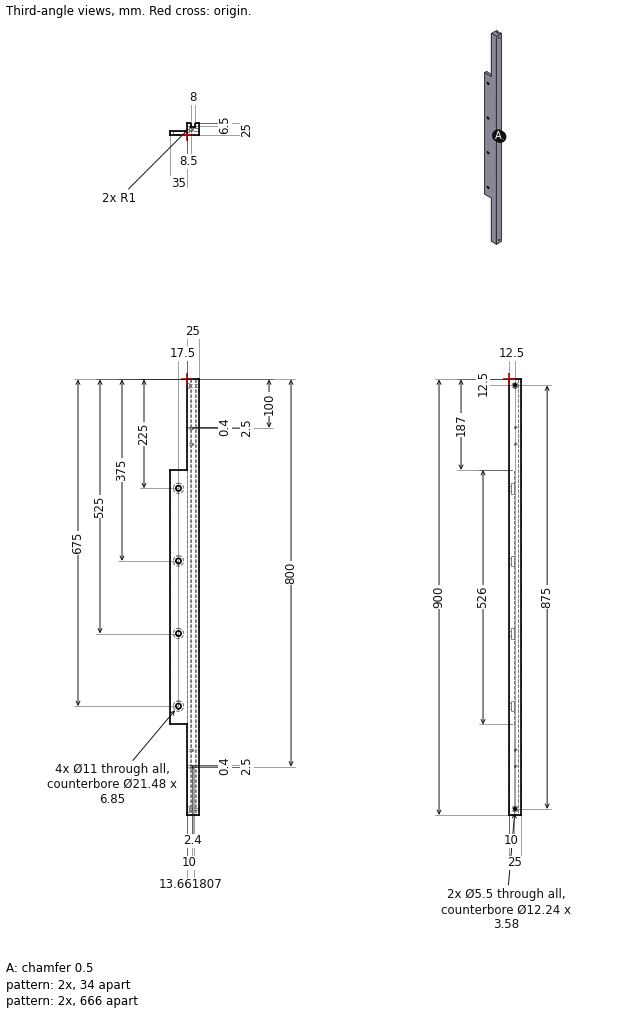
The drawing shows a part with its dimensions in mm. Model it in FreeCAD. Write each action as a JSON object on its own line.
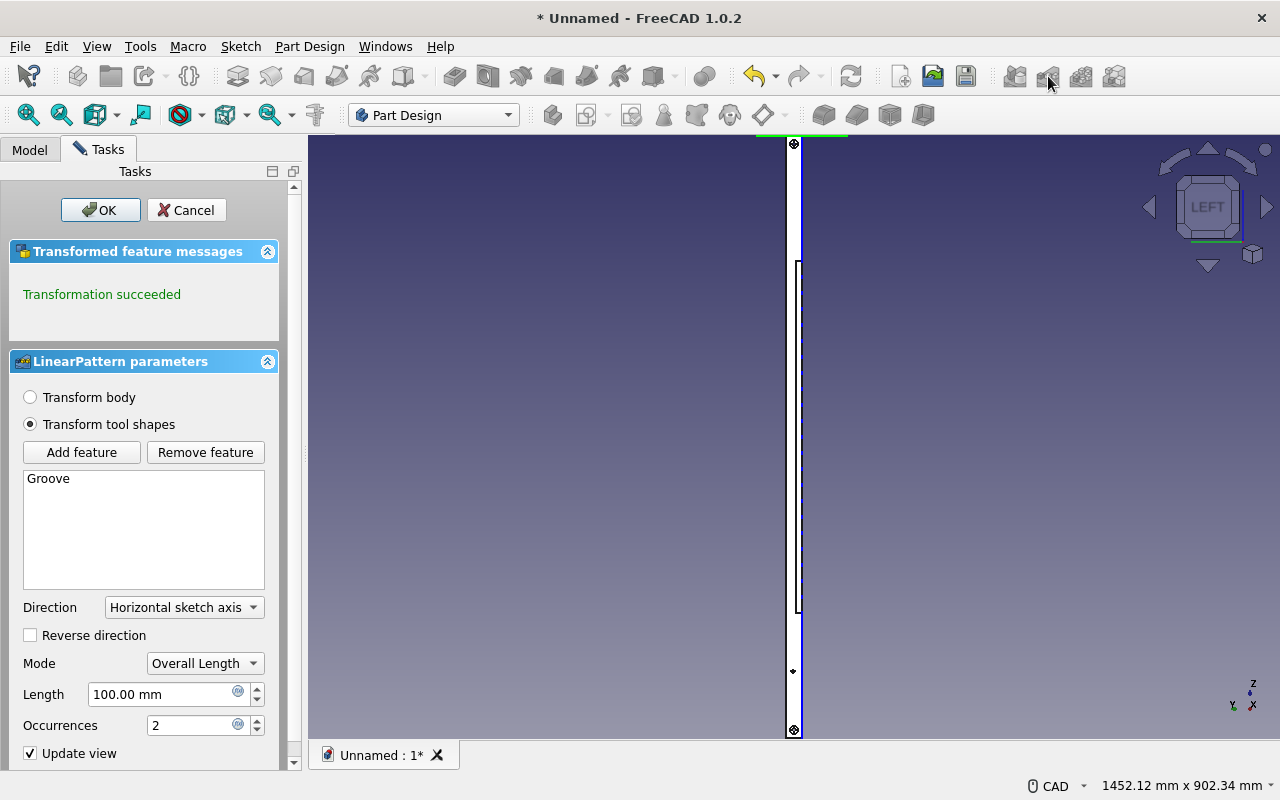
{"action": "left_click", "coordinate": [185, 608]}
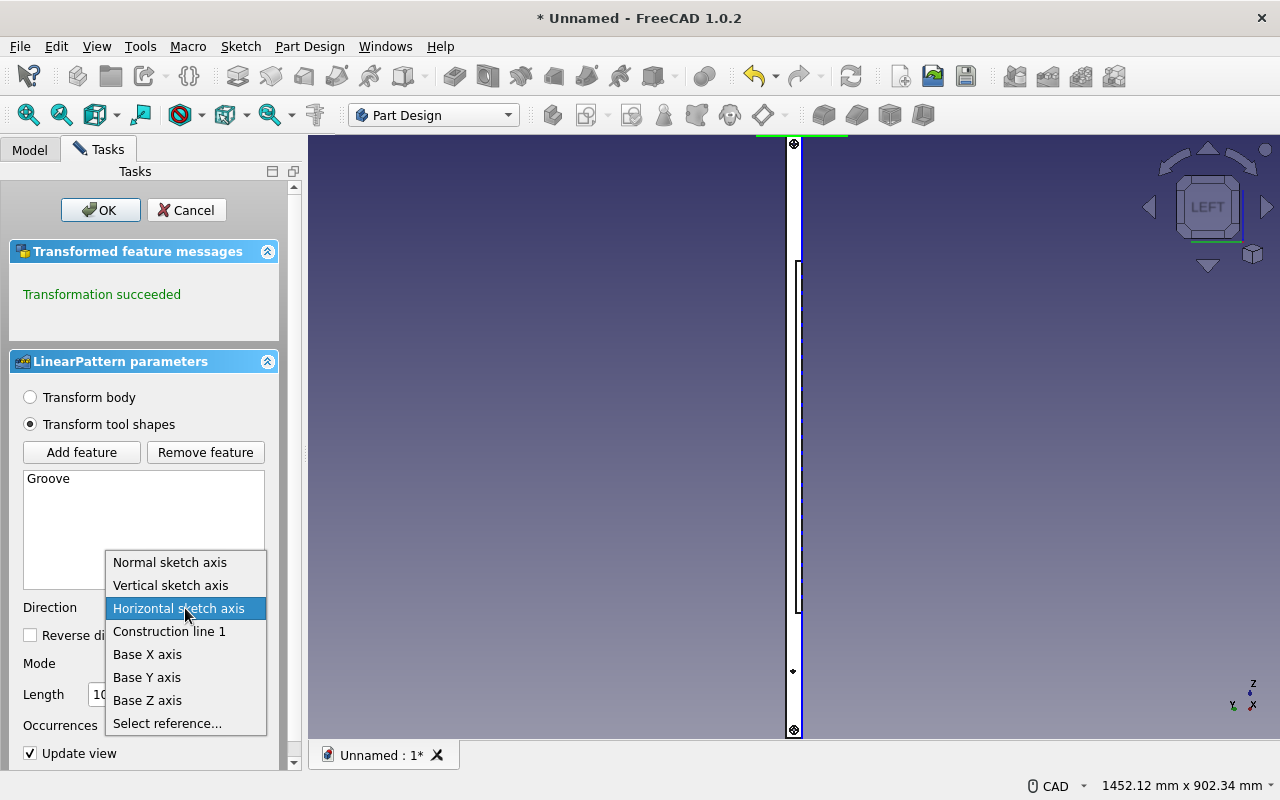
{"action": "left_click", "coordinate": [184, 700]}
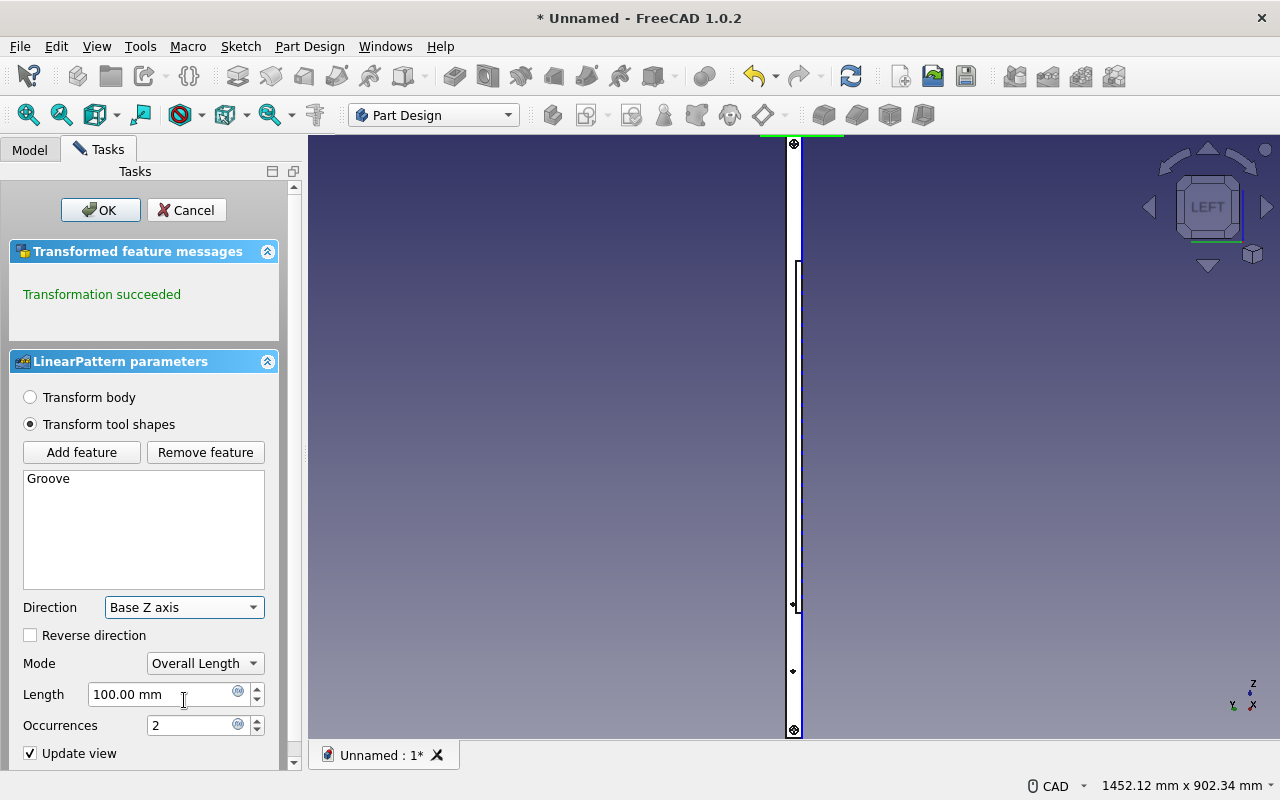
{"action": "left_click", "coordinate": [206, 664]}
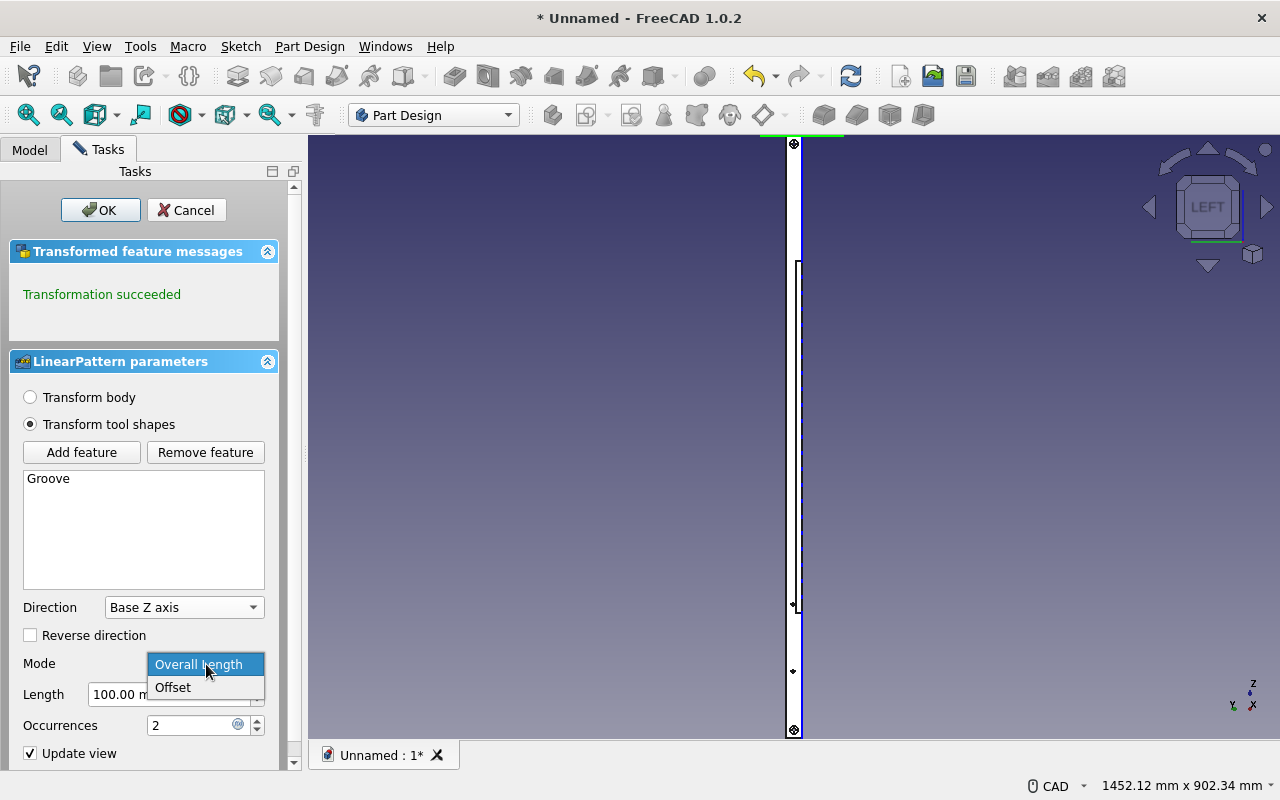
{"action": "left_click", "coordinate": [204, 688]}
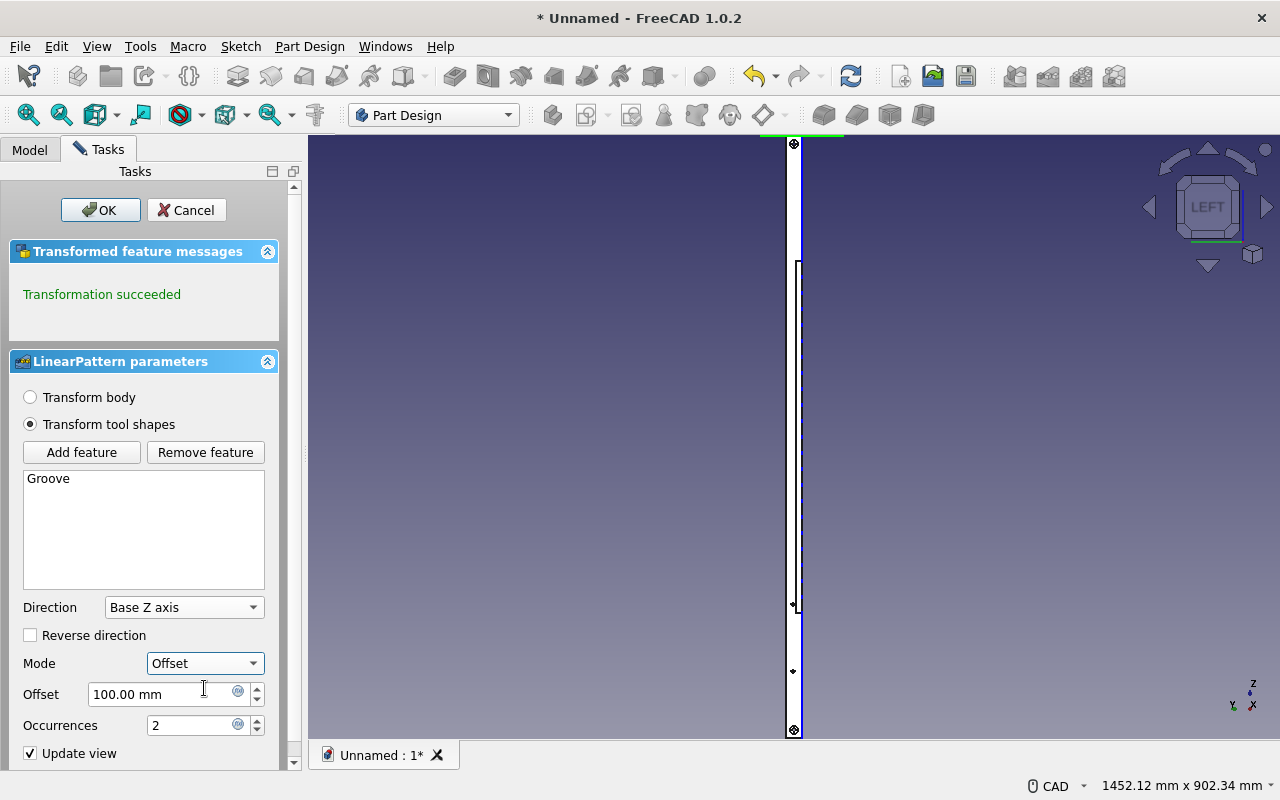
{"action": "triple_click", "coordinate": [170, 694]}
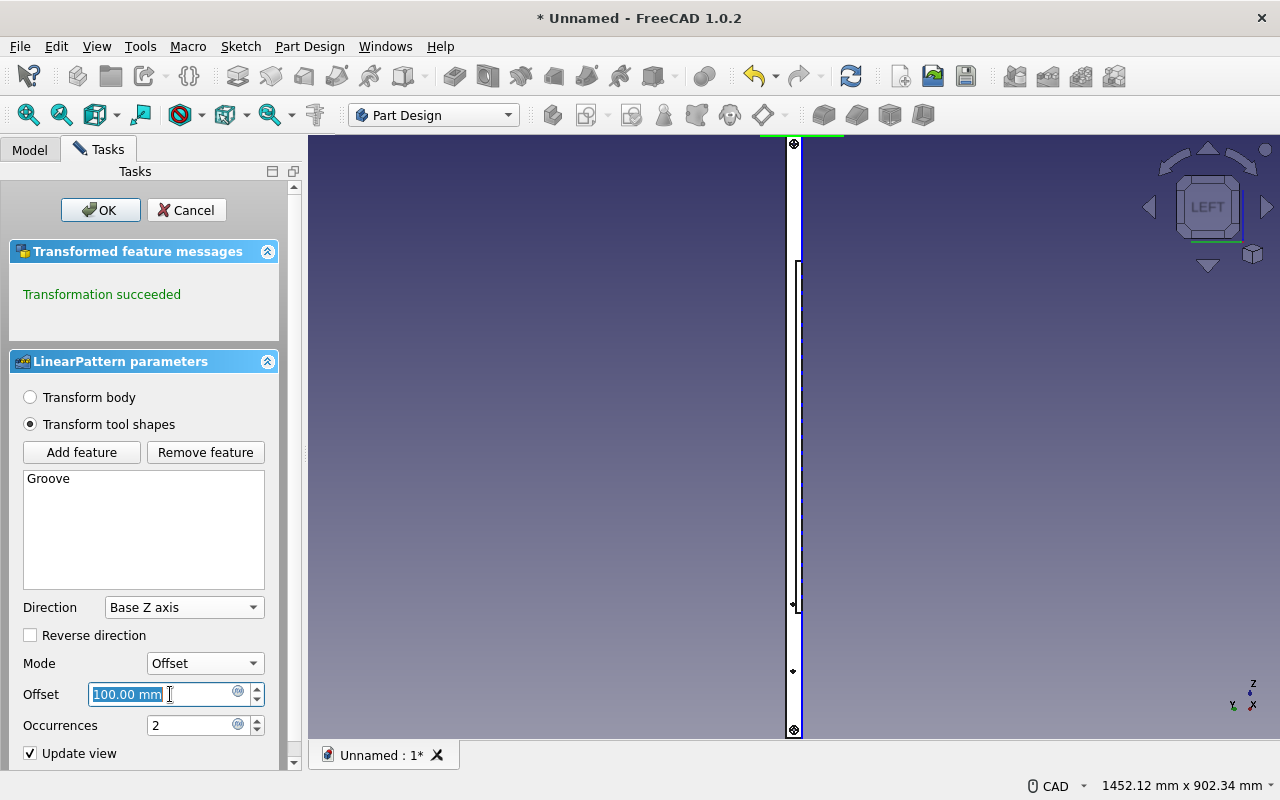
{"action": "type", "text": "34"}
{"action": "key", "text": "Tab"}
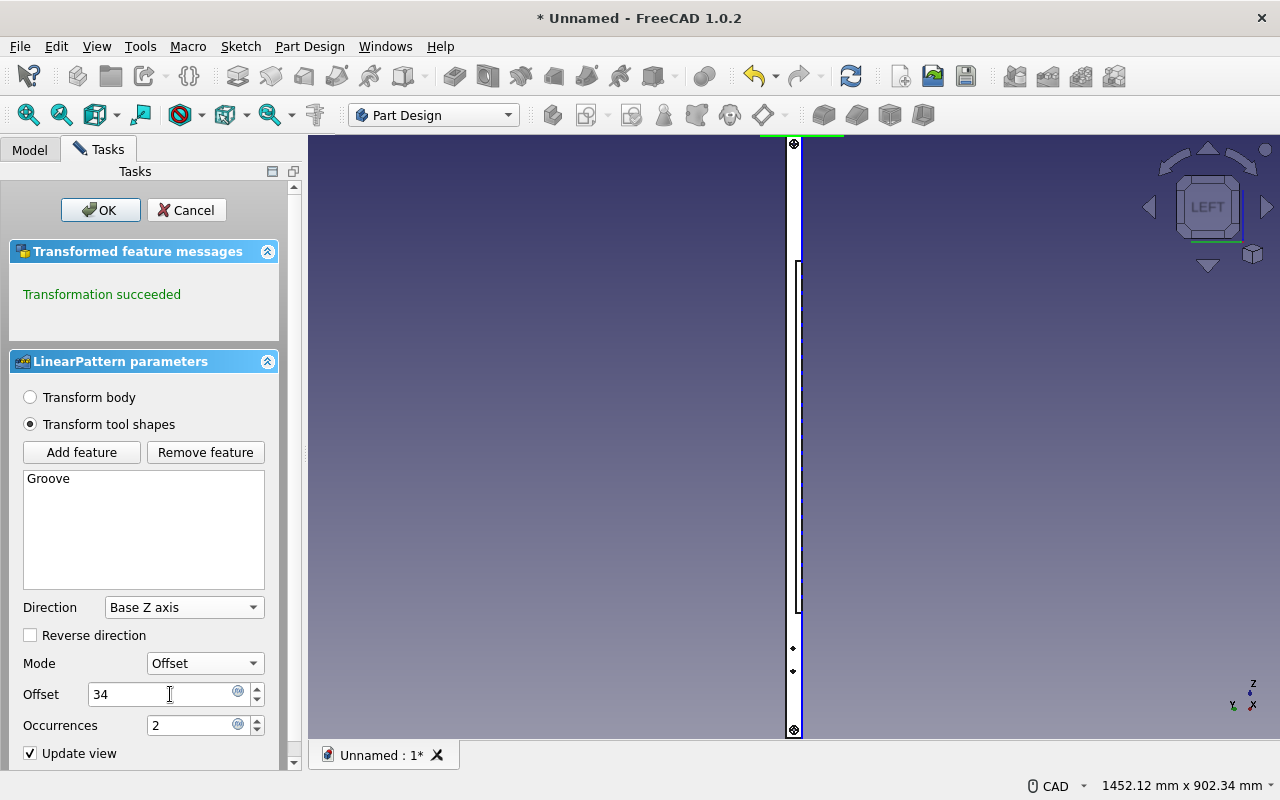
{"action": "triple_click", "coordinate": [199, 726]}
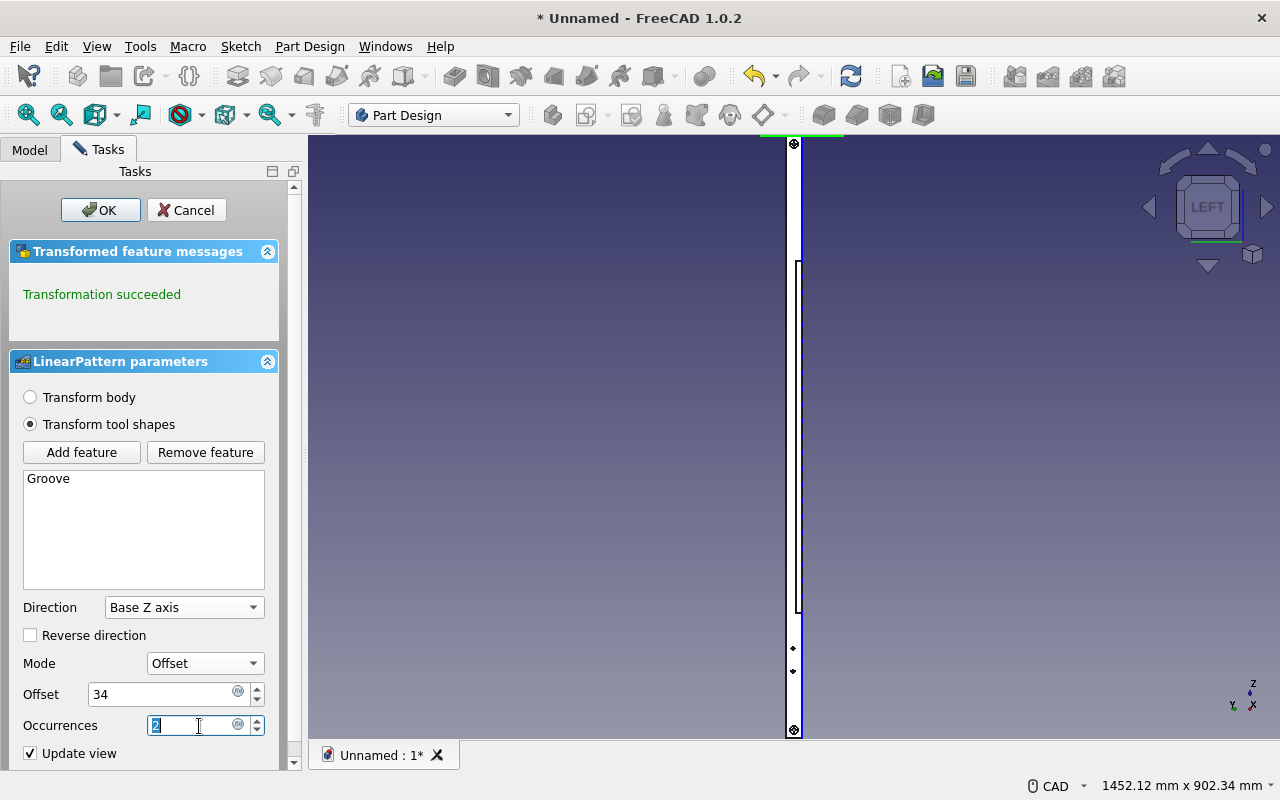
{"action": "type", "text": "2"}
{"action": "key", "text": "Tab"}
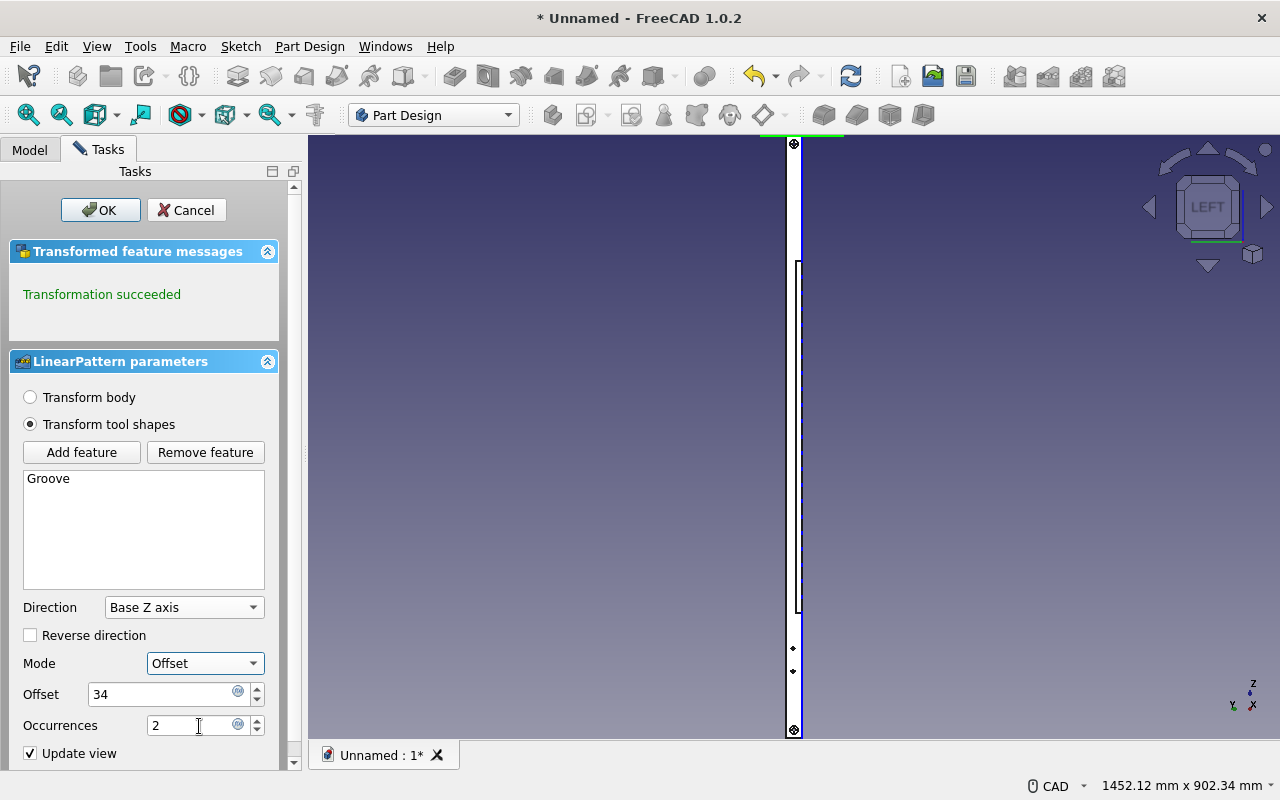
{"action": "left_click", "coordinate": [101, 210]}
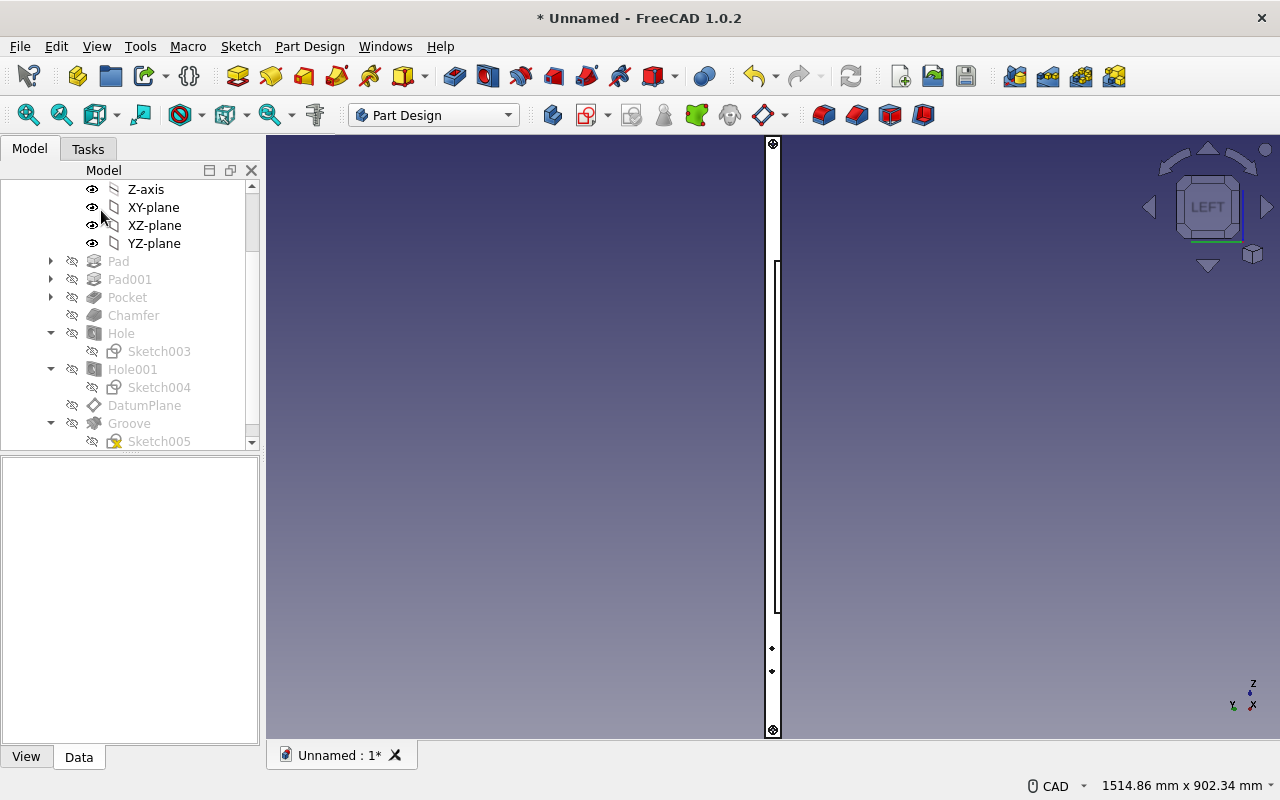
{"action": "left_click", "coordinate": [117, 423]}